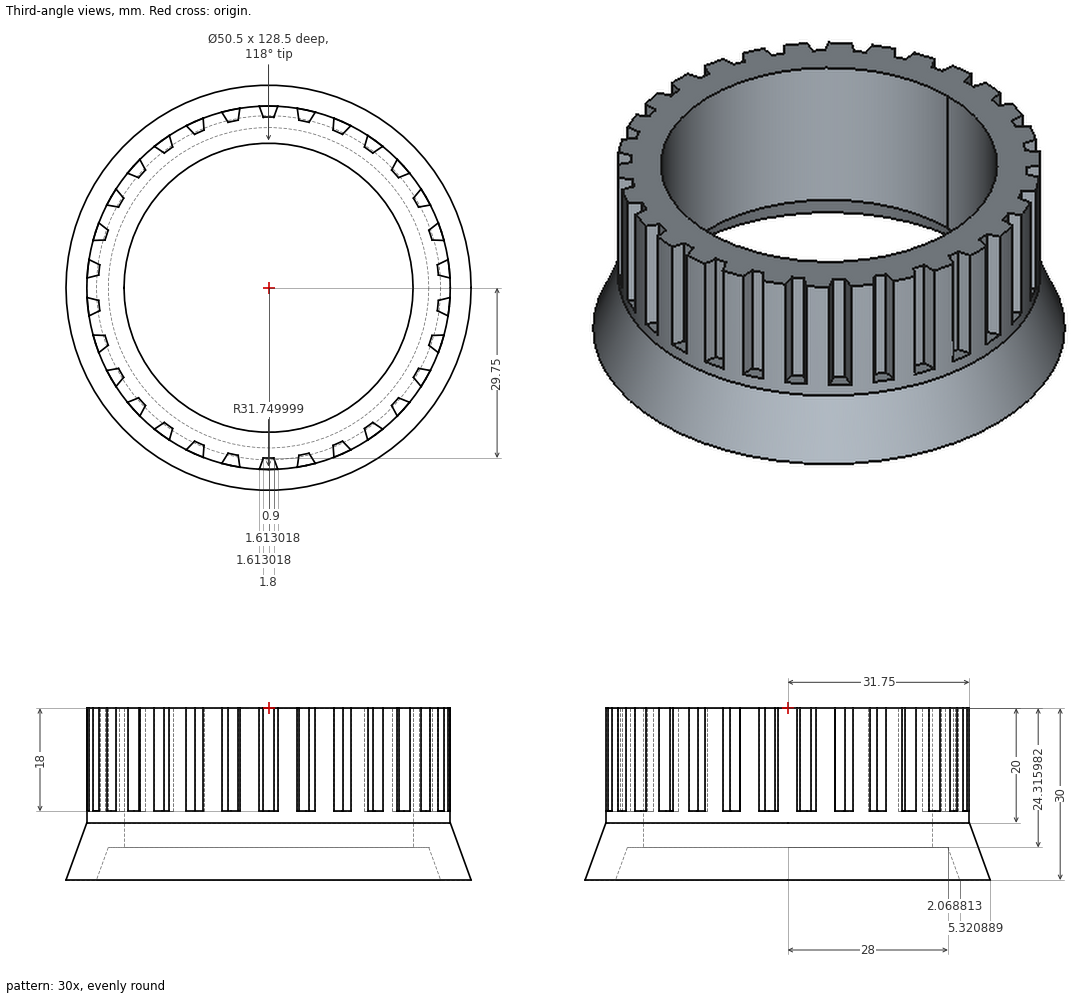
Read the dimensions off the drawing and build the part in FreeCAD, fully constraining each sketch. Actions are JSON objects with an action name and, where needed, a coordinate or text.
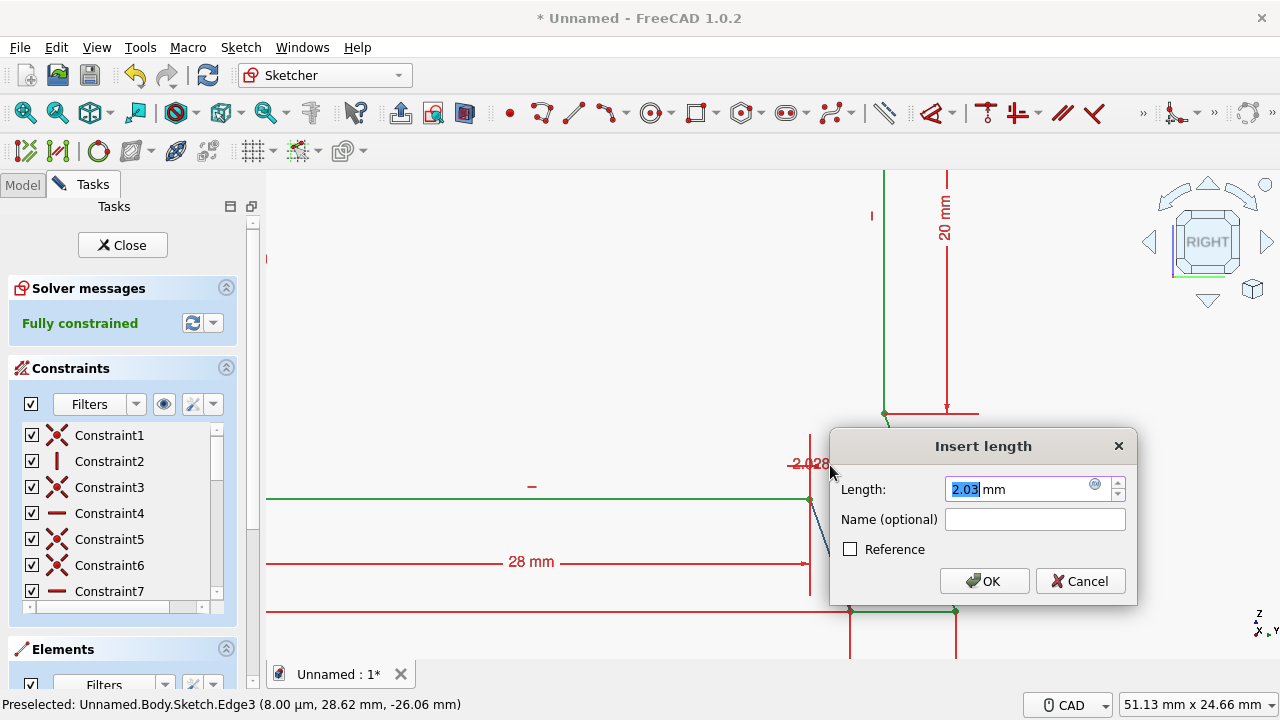
{"action": "type", "text": "2.068813"}
{"action": "key", "text": "Return"}
{"action": "key", "text": "Escape"}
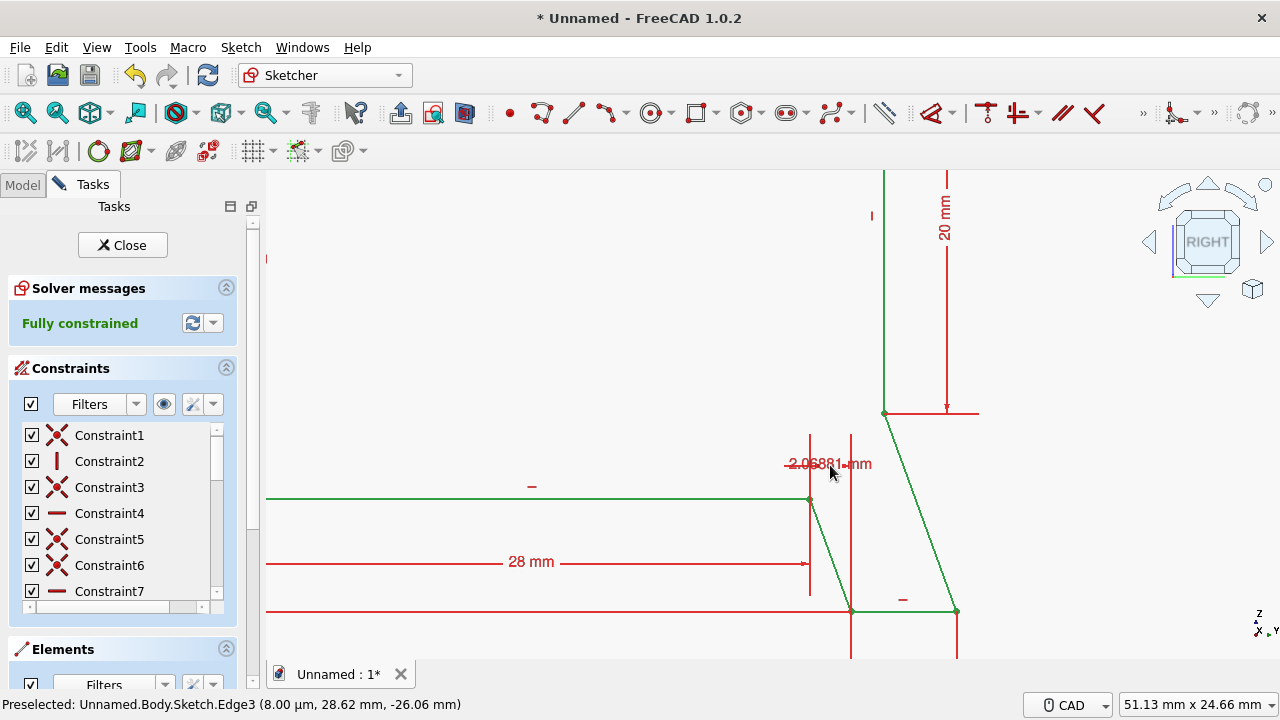
{"action": "left_click", "coordinate": [123, 245]}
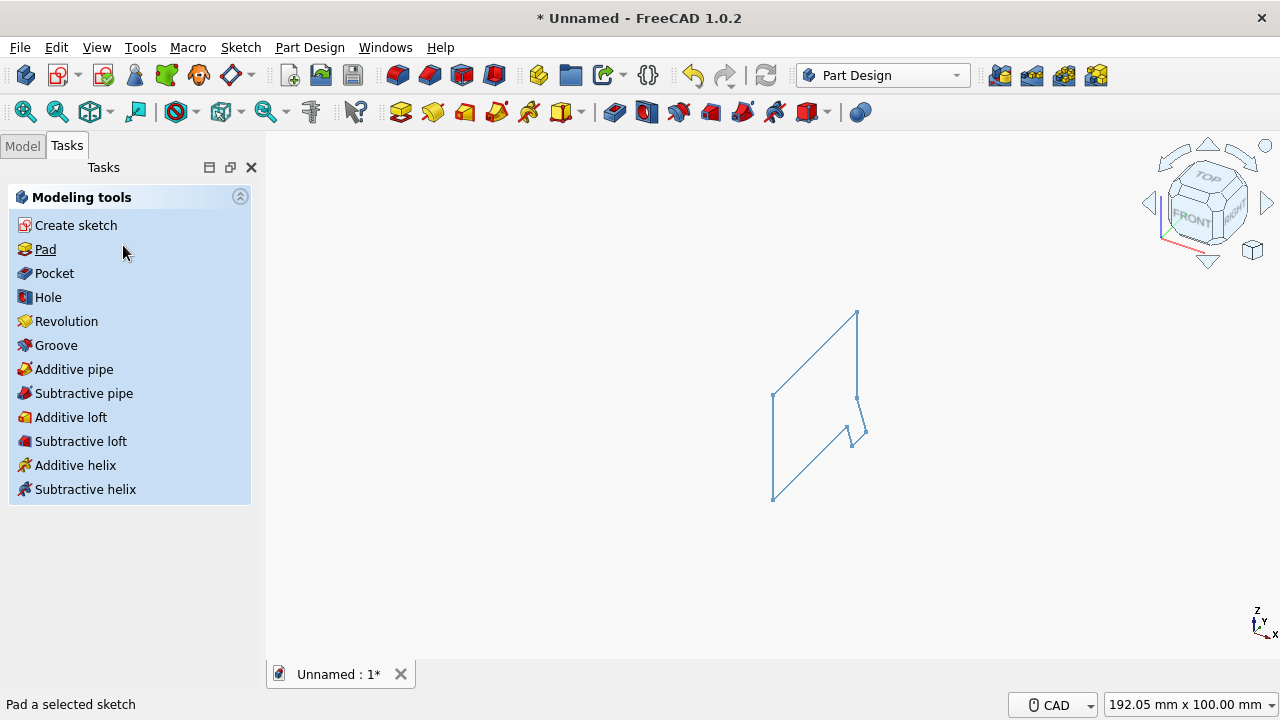
{"action": "left_click", "coordinate": [434, 112]}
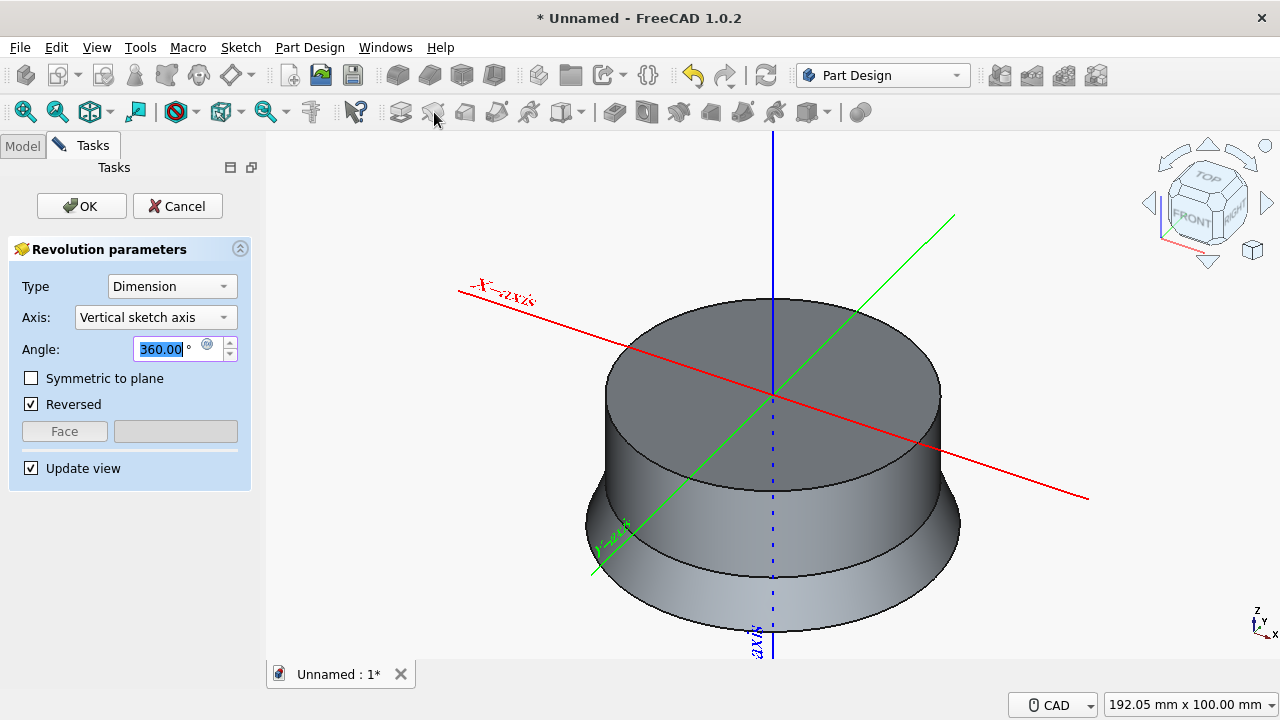
{"action": "left_click", "coordinate": [82, 206]}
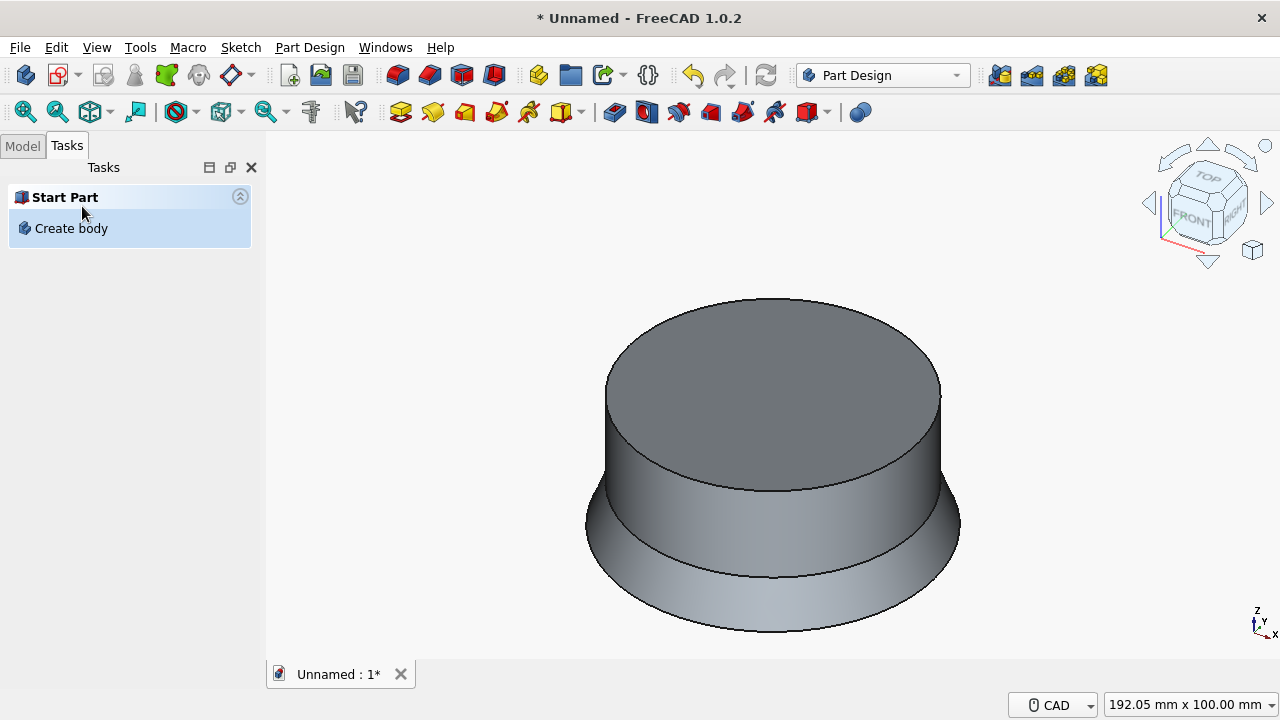
{"action": "key", "text": "v f"}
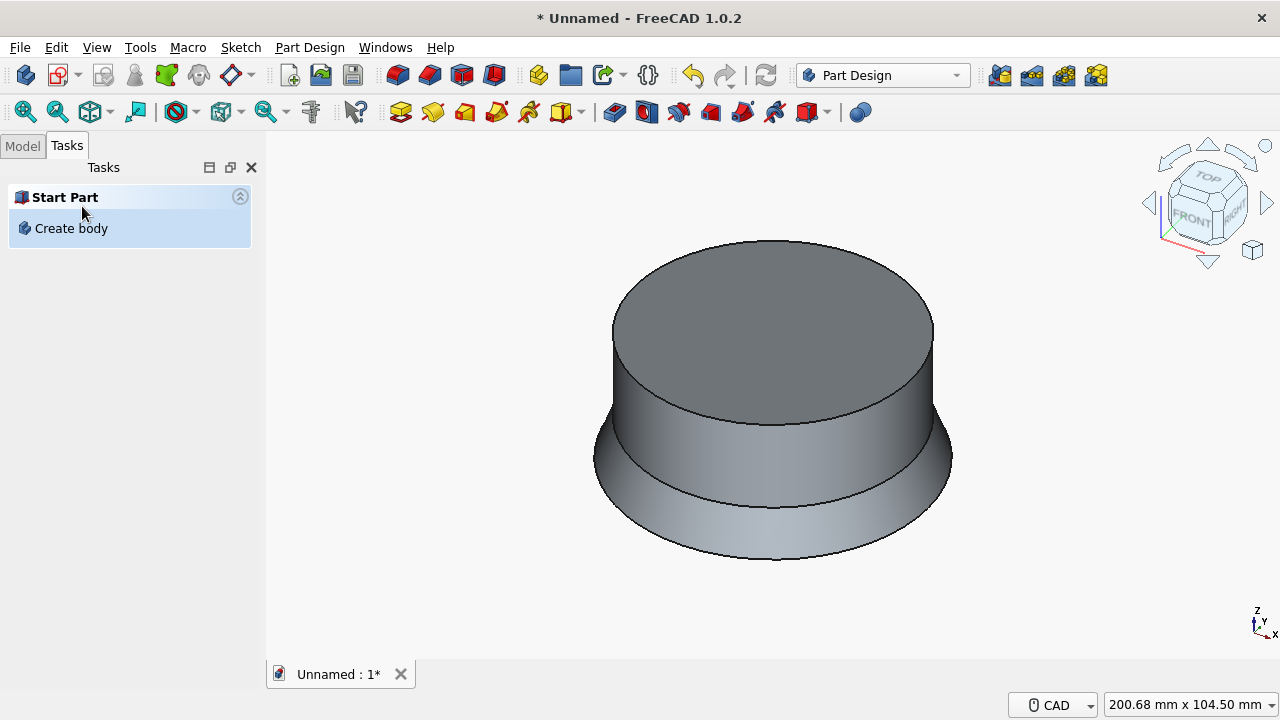
{"action": "left_click", "coordinate": [58, 76]}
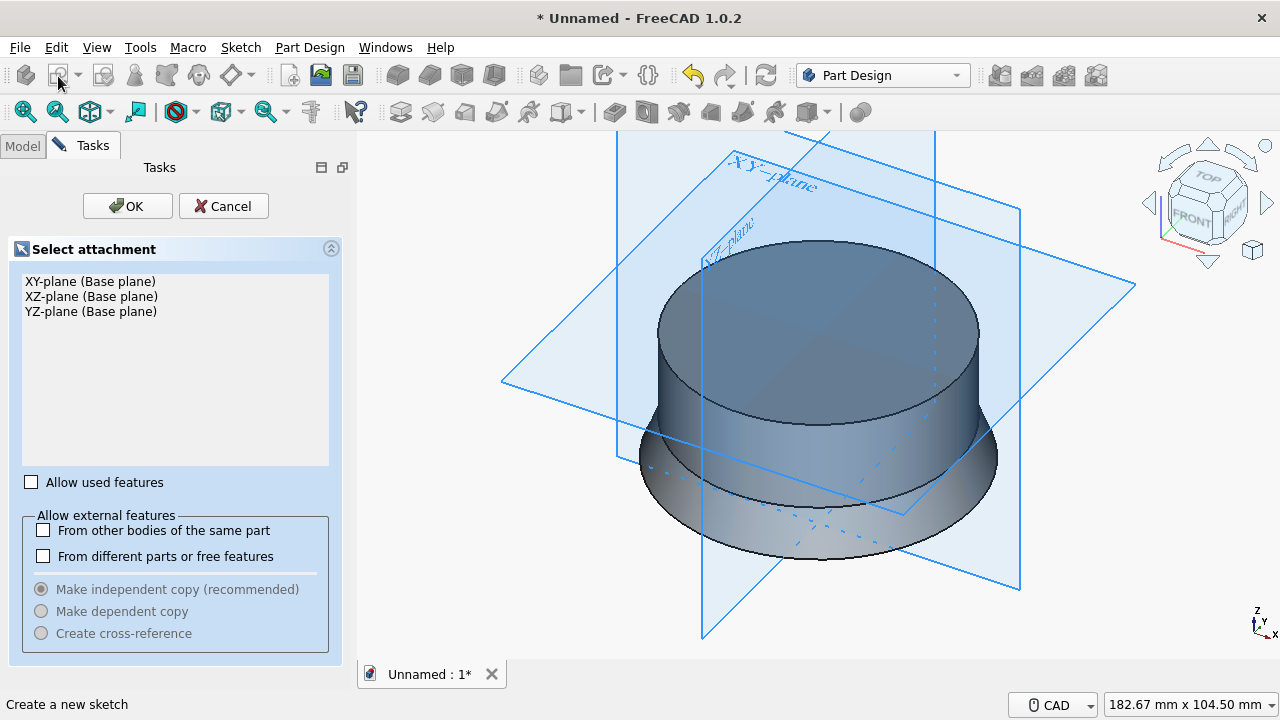
{"action": "left_click", "coordinate": [82, 282]}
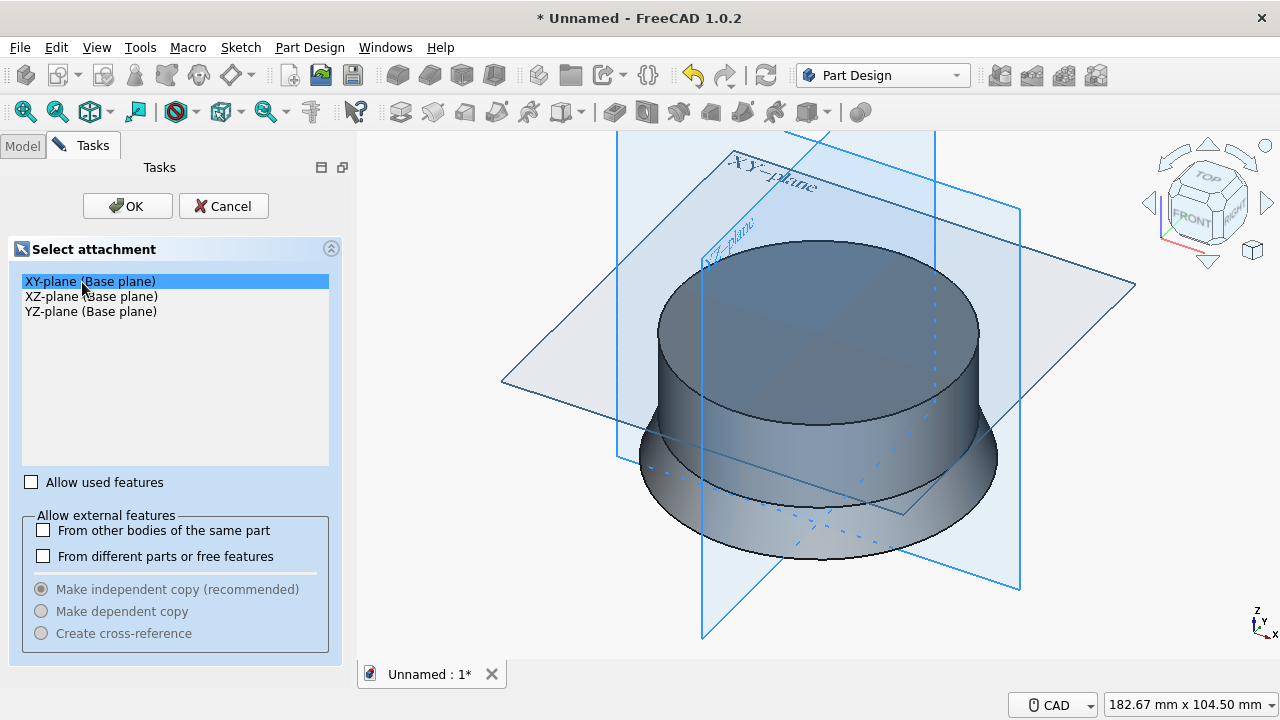
{"action": "left_click", "coordinate": [128, 206]}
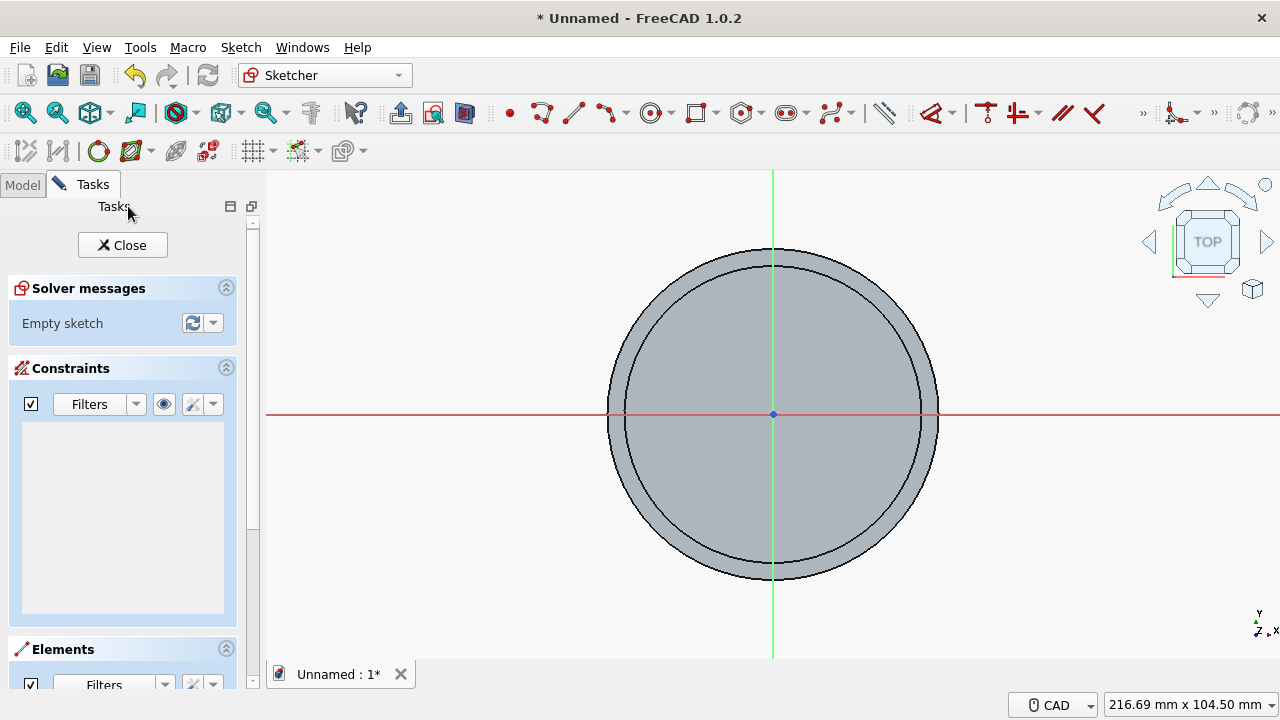
{"action": "left_click", "coordinate": [652, 114]}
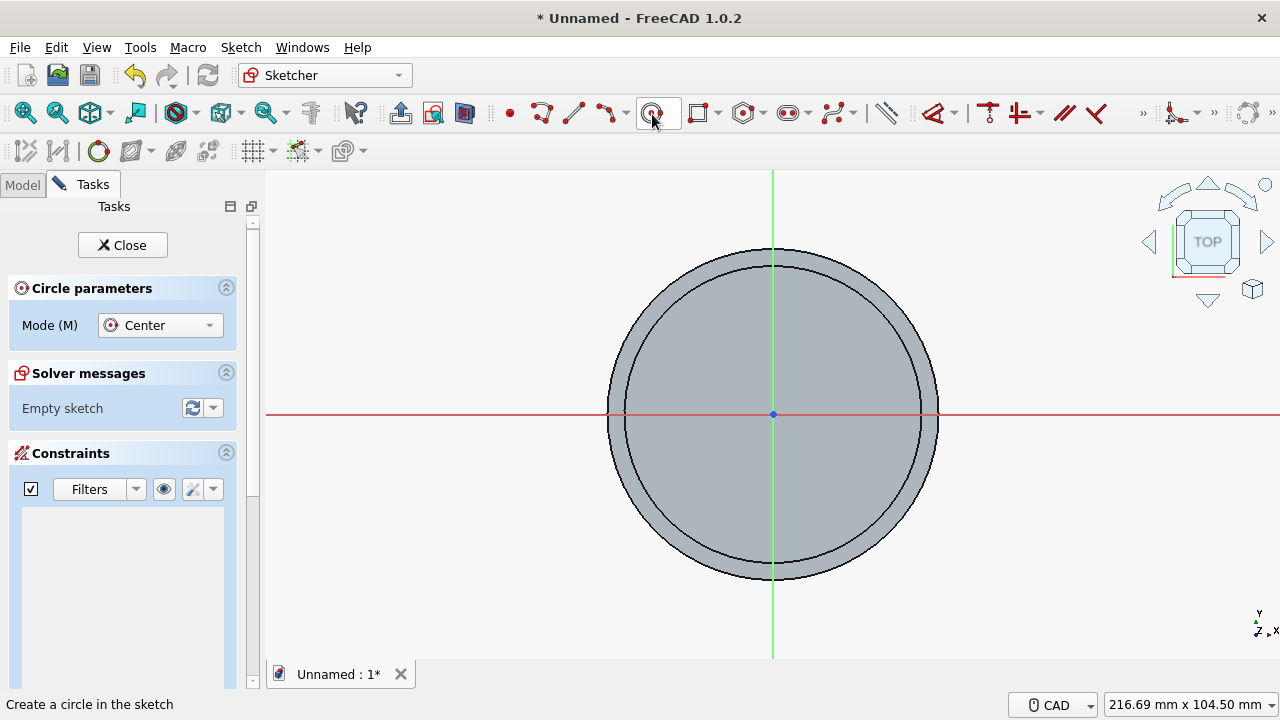
{"action": "left_click", "coordinate": [773, 414]}
{"action": "mouse_move", "coordinate": [857, 331]}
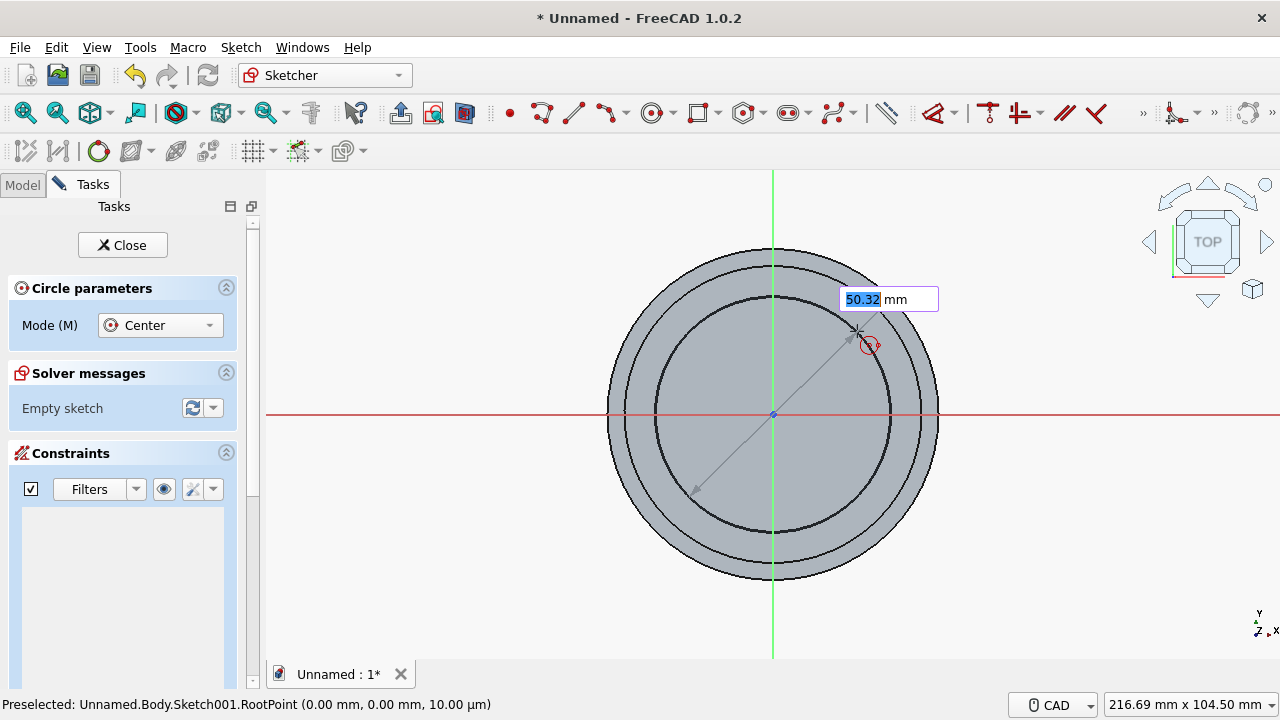
{"action": "type", "text": "50.5"}
{"action": "key", "text": "Return"}
{"action": "key", "text": "Escape"}